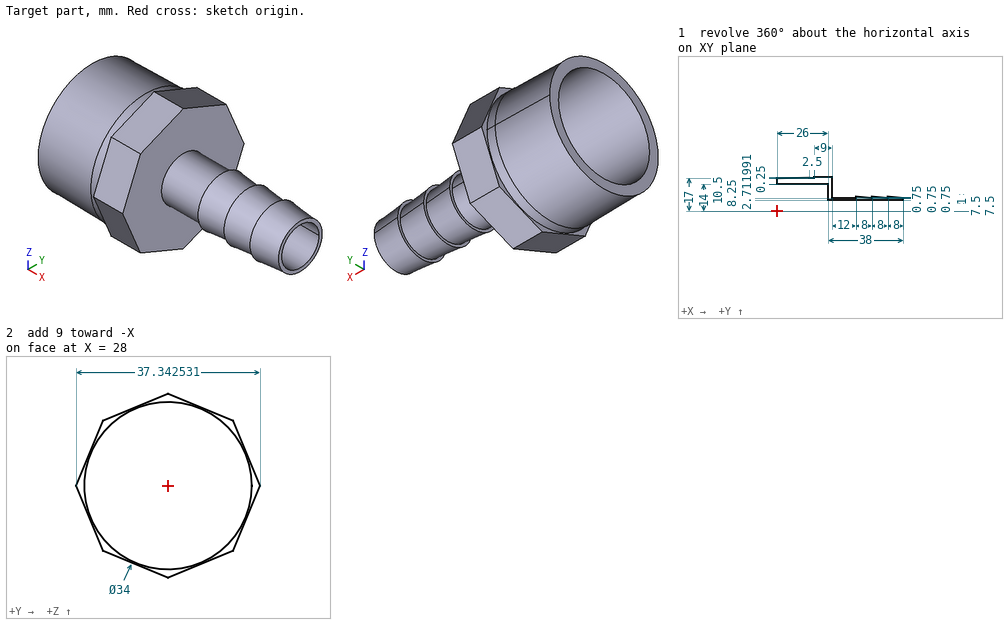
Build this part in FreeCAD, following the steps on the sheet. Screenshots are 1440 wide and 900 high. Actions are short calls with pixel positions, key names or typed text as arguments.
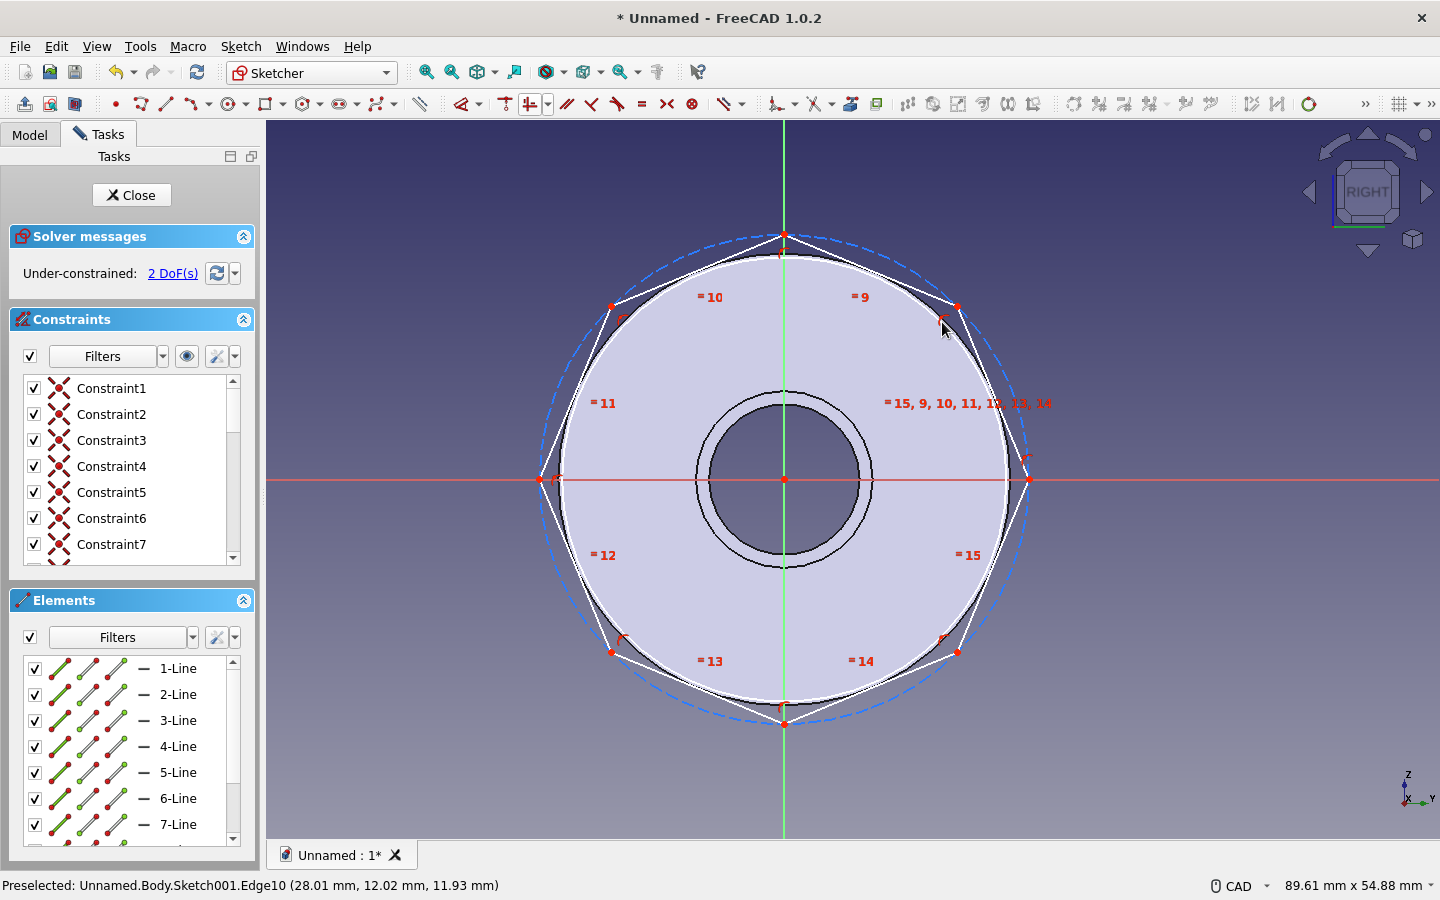
click(460, 104)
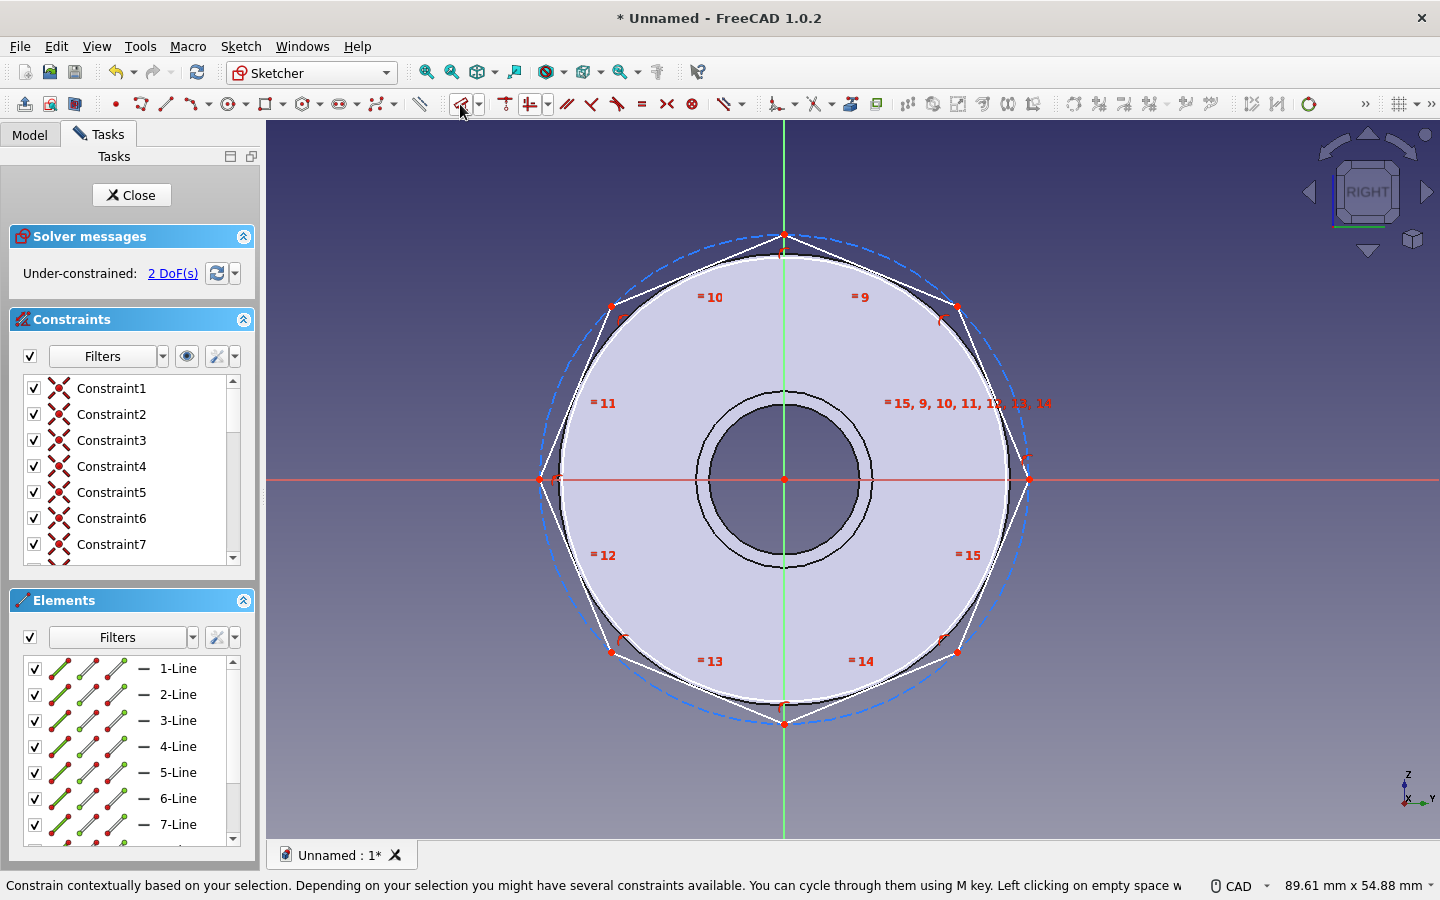
click(941, 322)
click(980, 283)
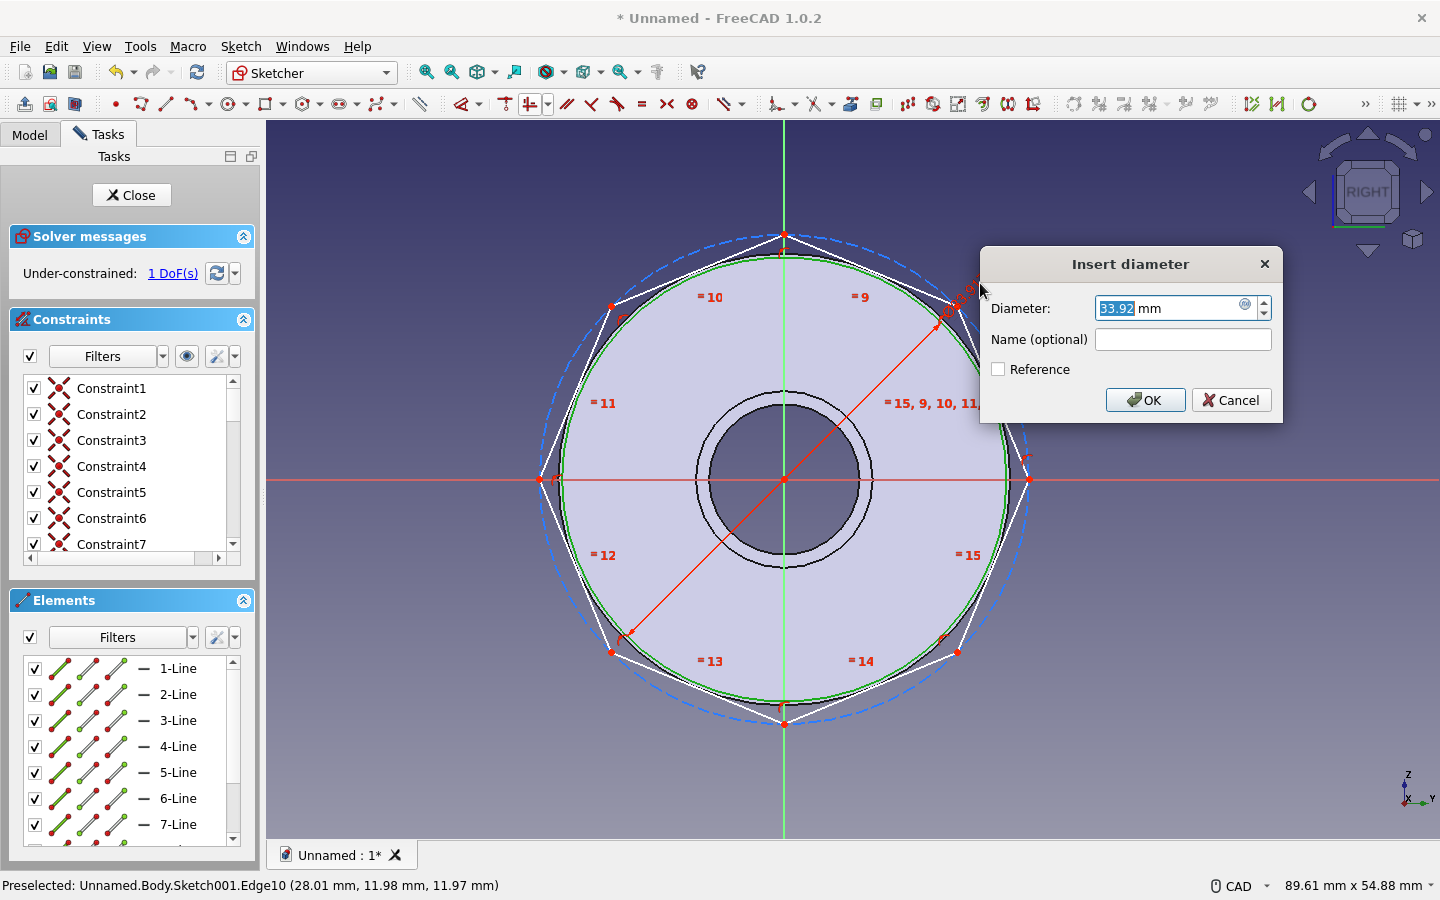
text(34)
key(Return)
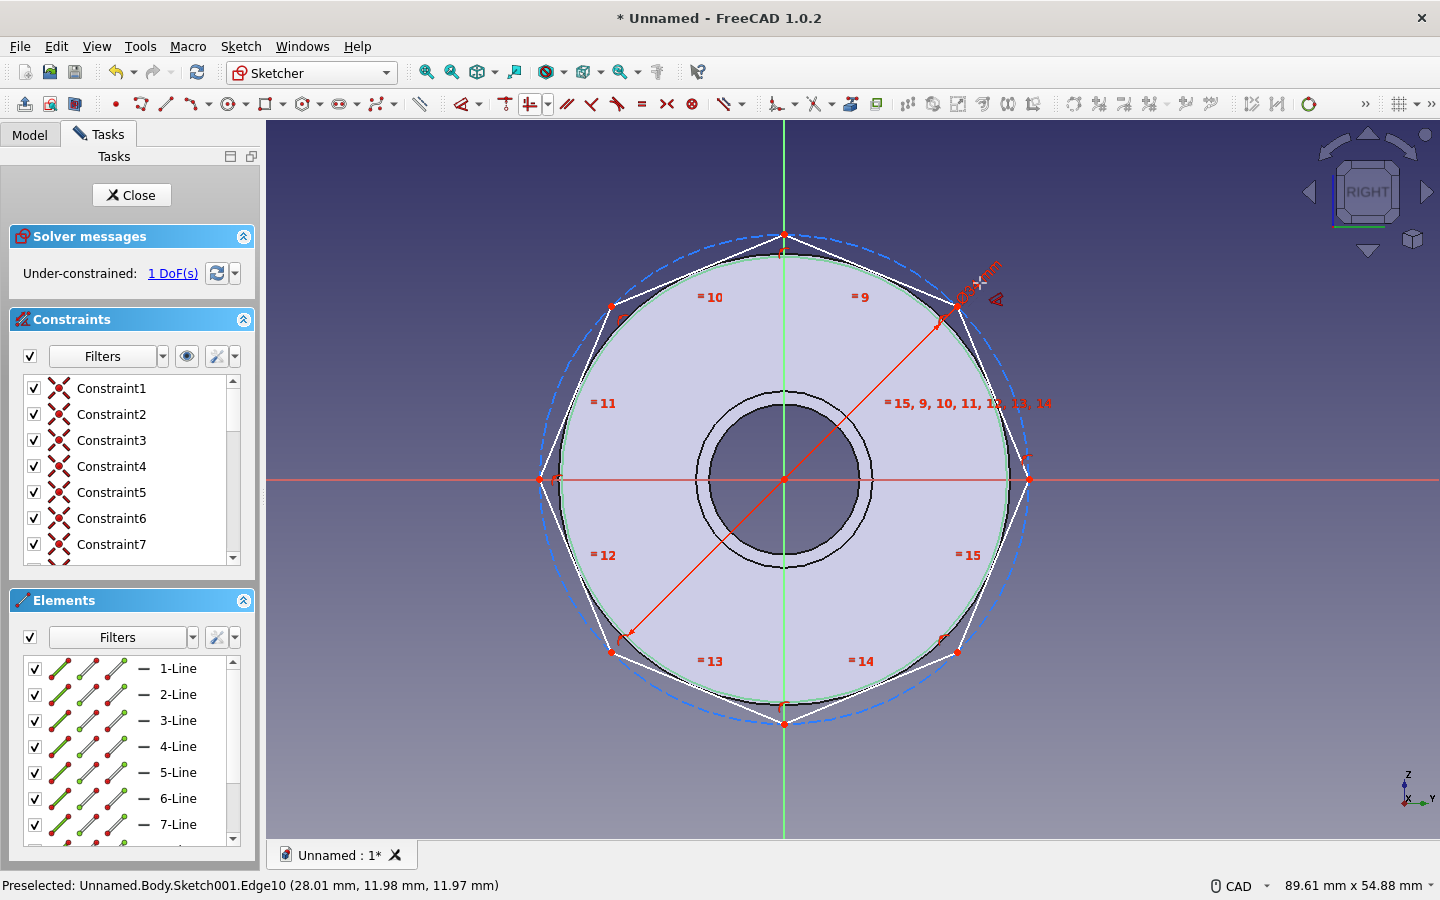
click(540, 479)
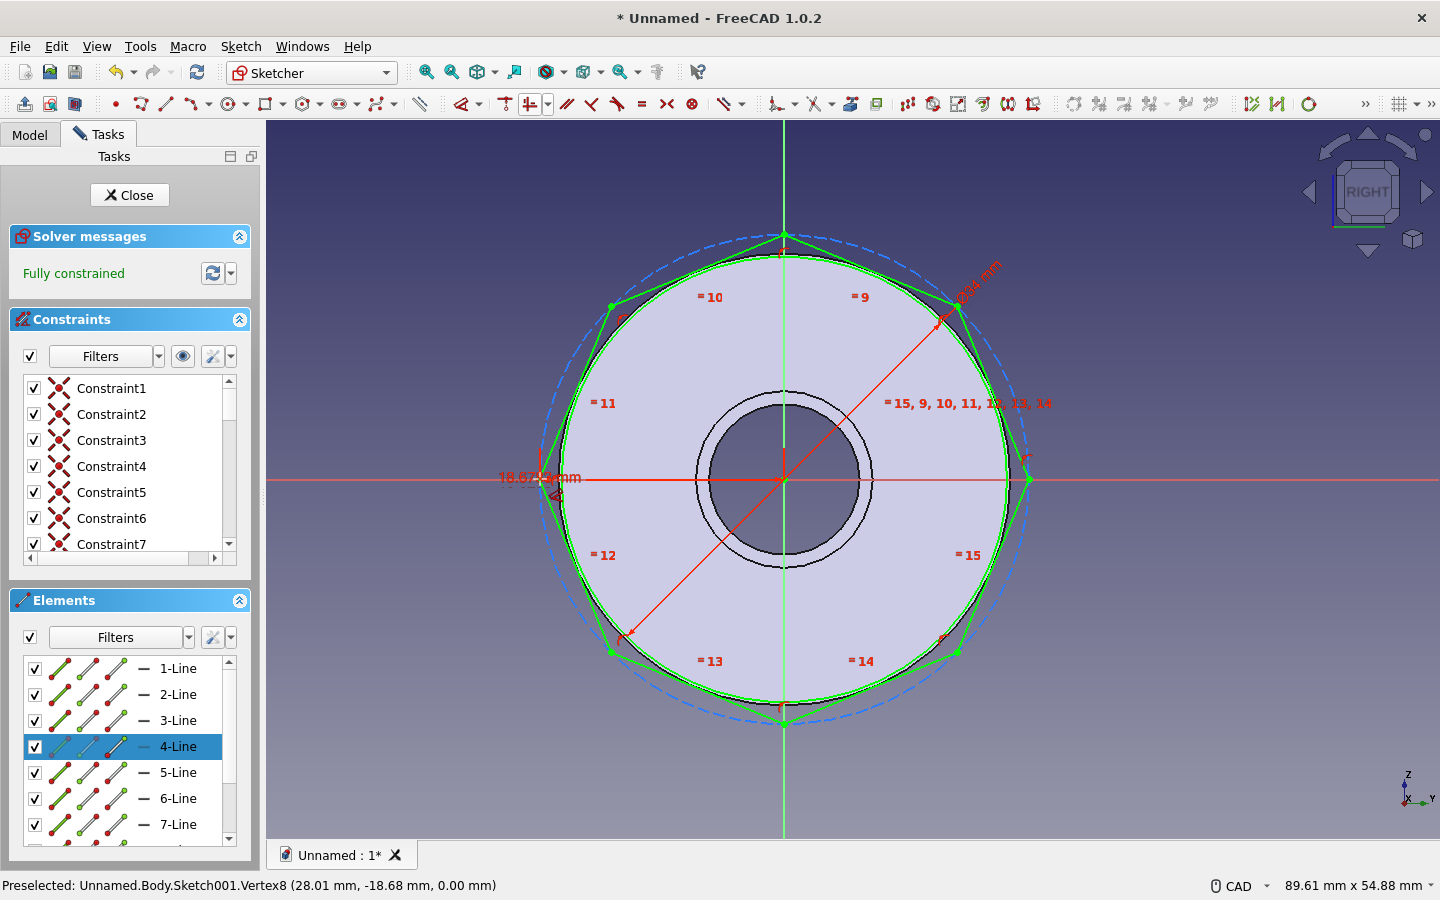
click(1029, 479)
click(672, 513)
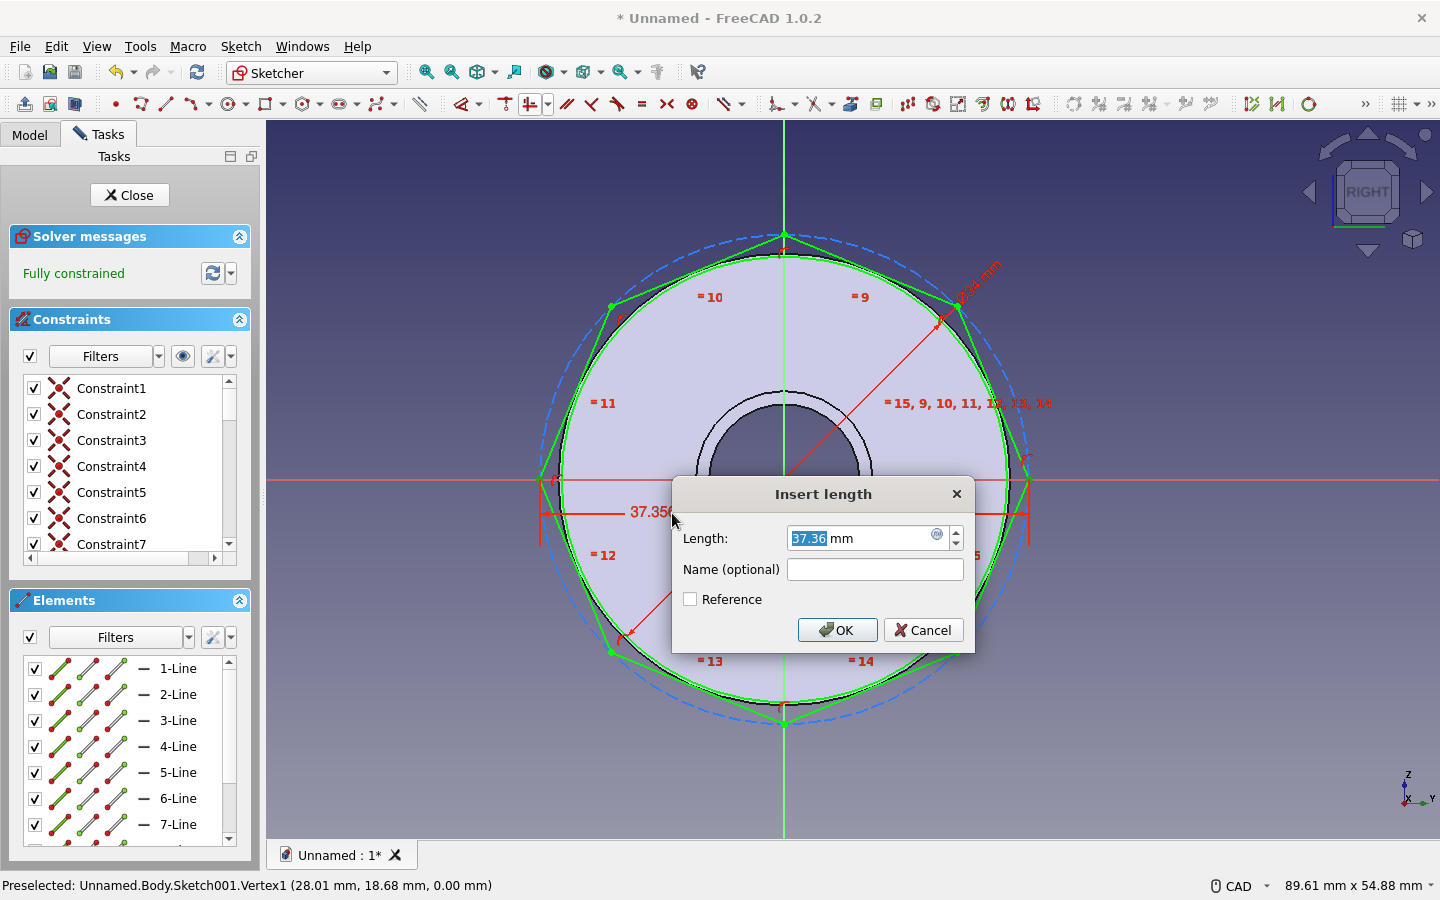
text(37.342531)
key(Return)
key(Escape)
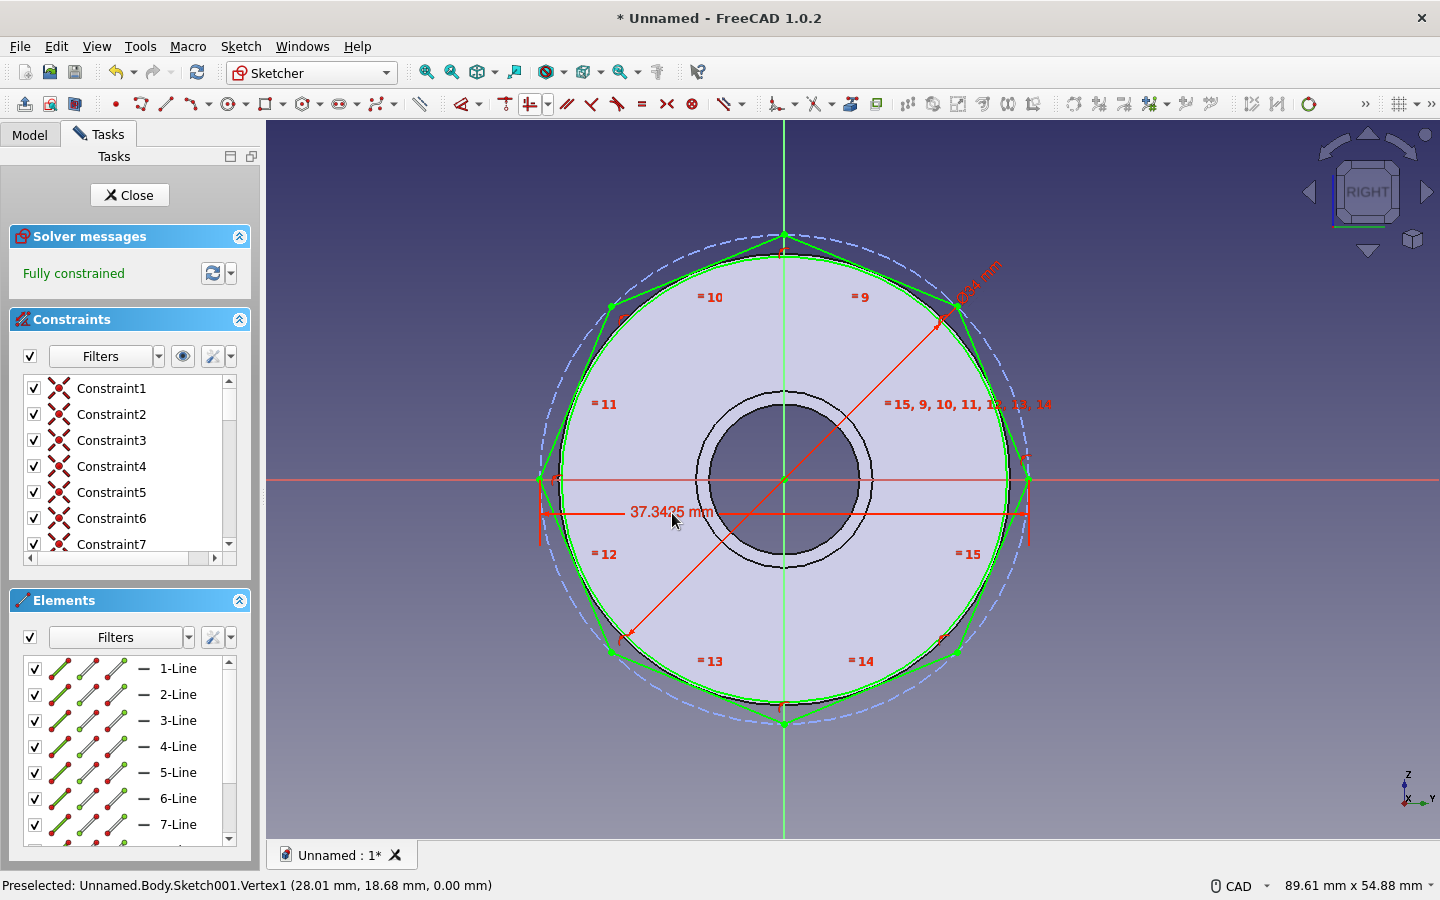
click(130, 195)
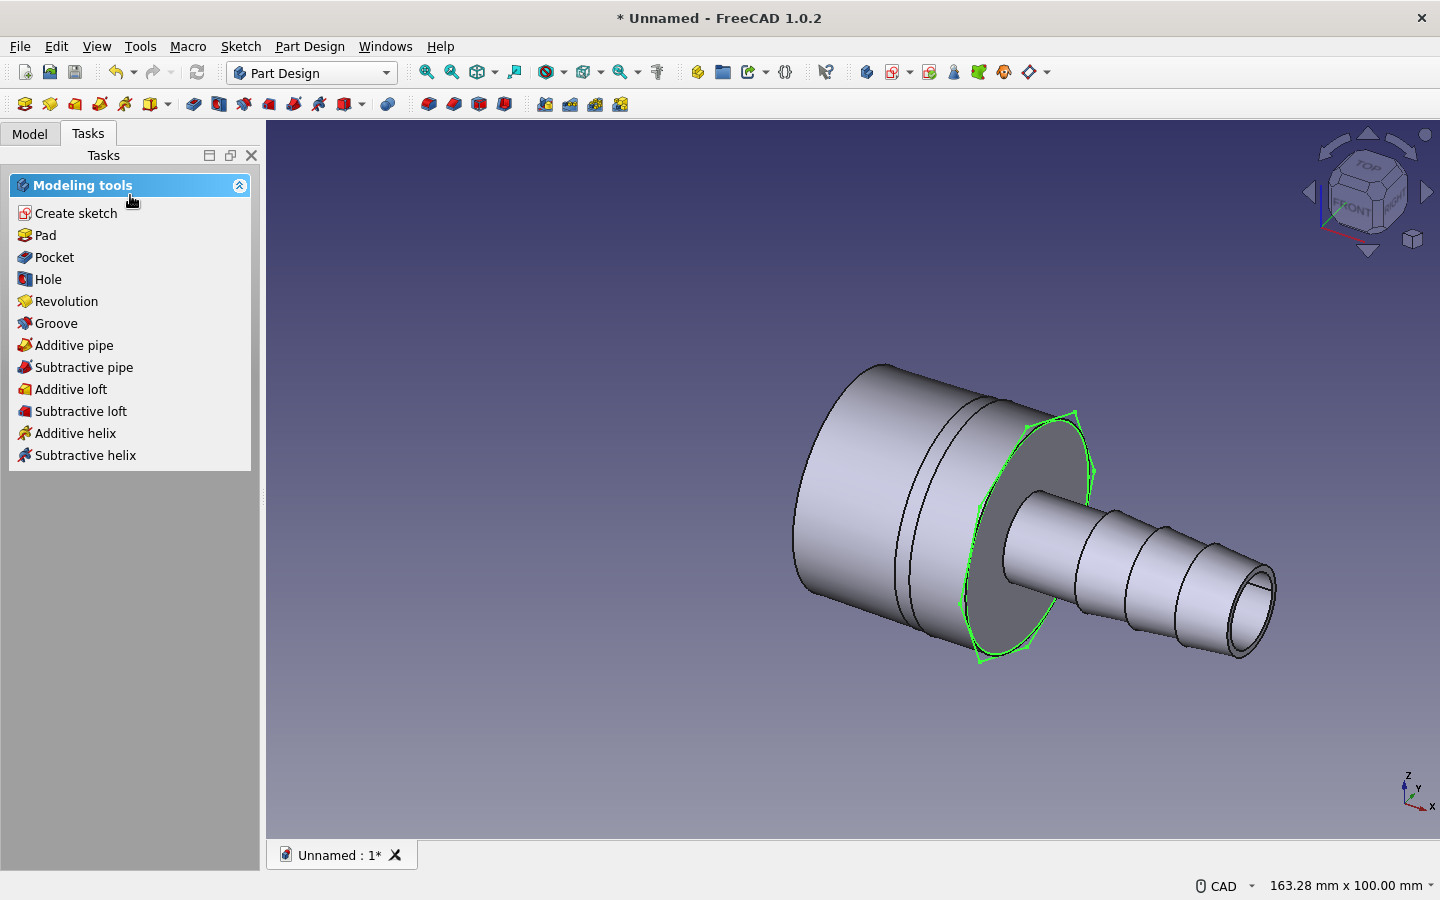
click(25, 104)